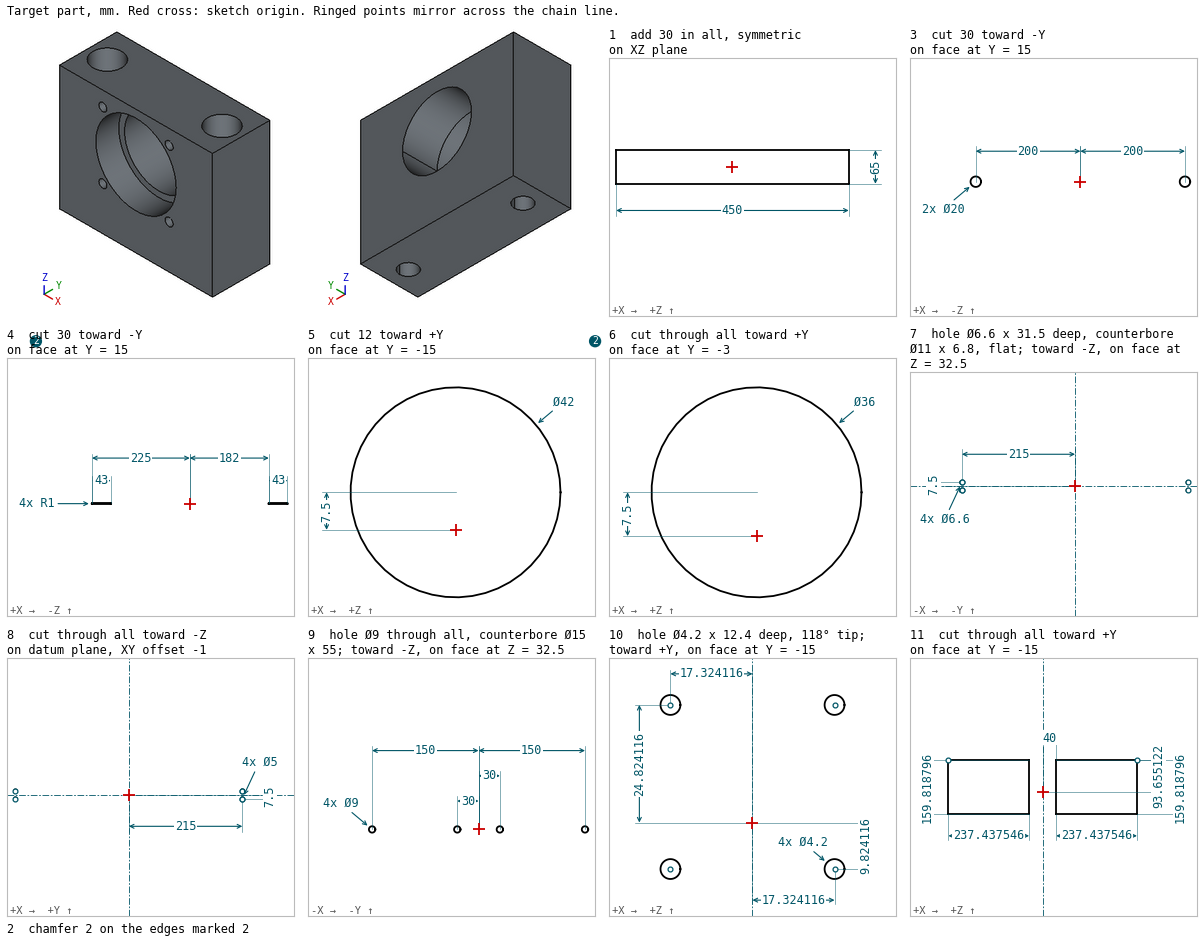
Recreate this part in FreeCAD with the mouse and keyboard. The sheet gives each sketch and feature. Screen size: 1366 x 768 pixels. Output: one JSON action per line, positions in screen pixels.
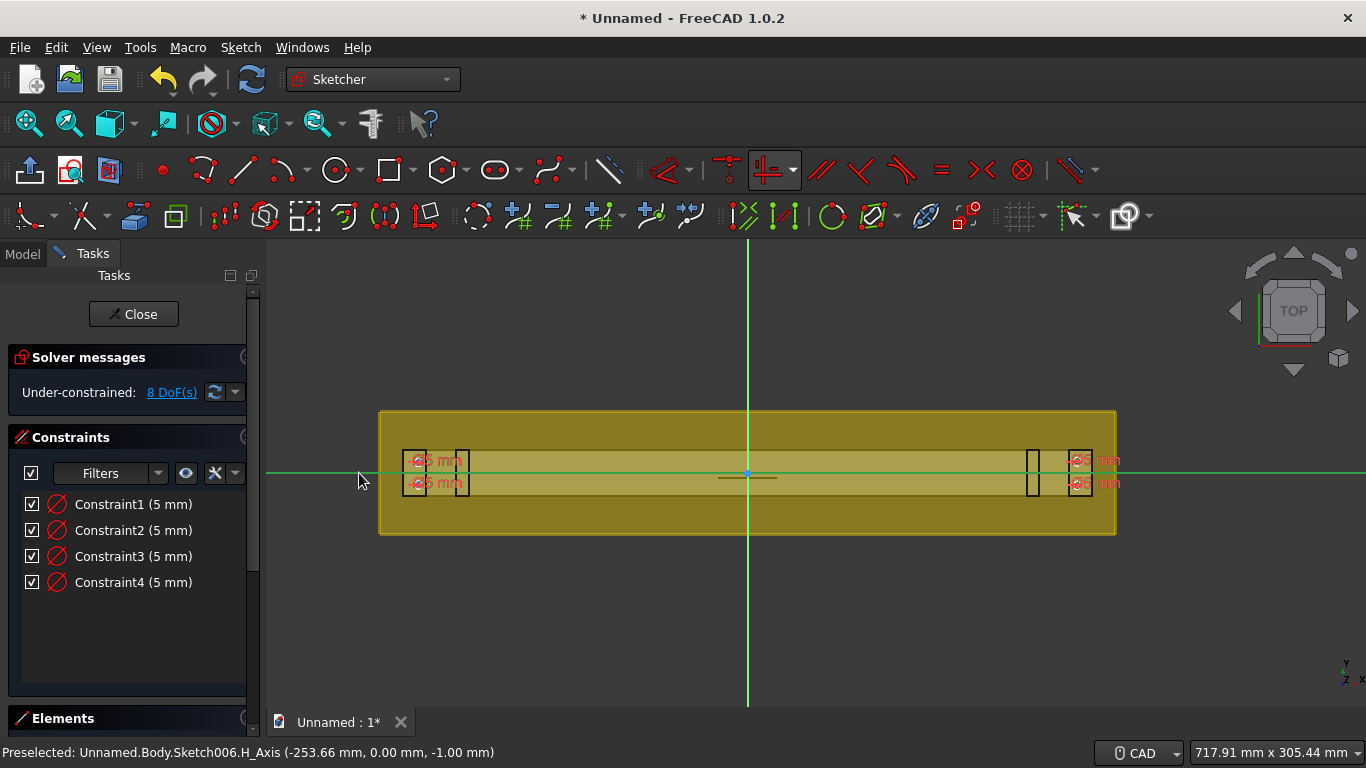
{"action": "key", "text": "s"}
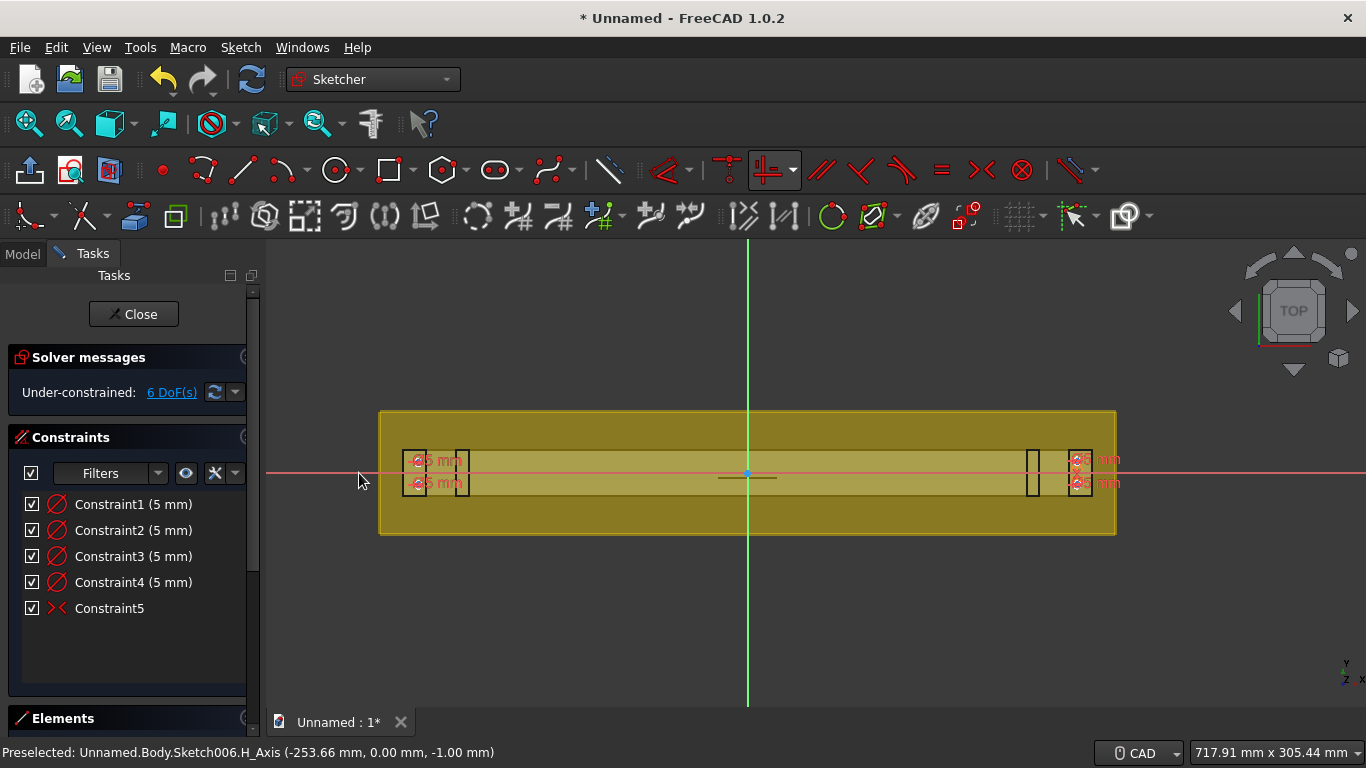
{"action": "left_click", "coordinate": [1077, 485]}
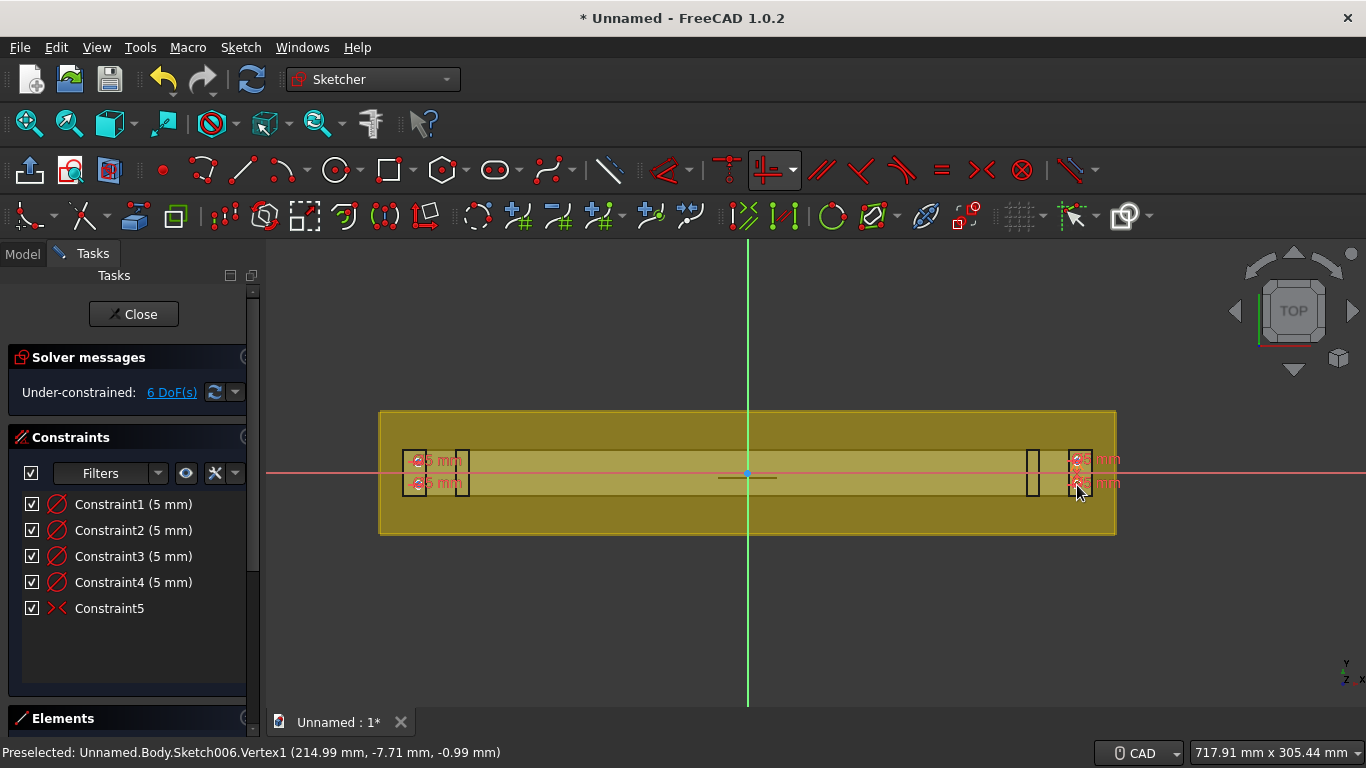
{"action": "left_click", "coordinate": [419, 485]}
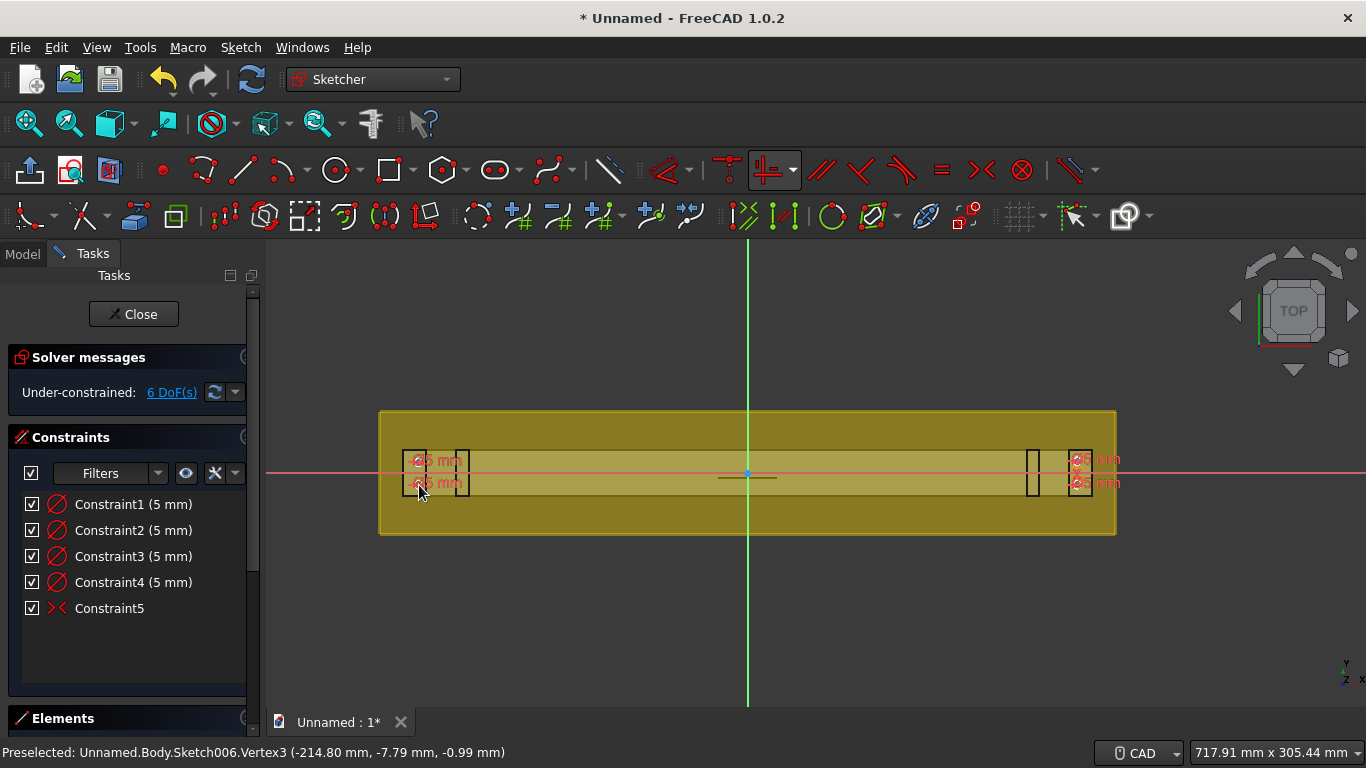
{"action": "left_click", "coordinate": [748, 650]}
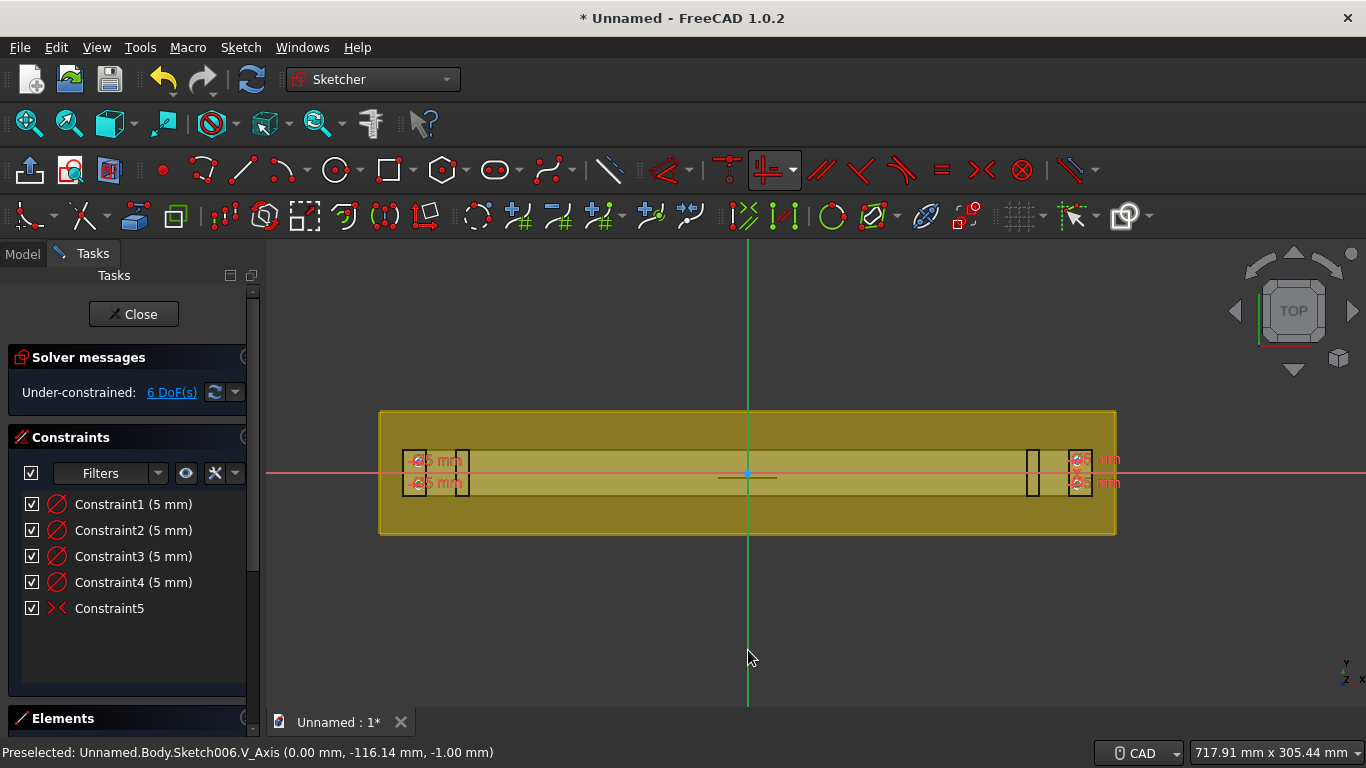
{"action": "left_click", "coordinate": [982, 170]}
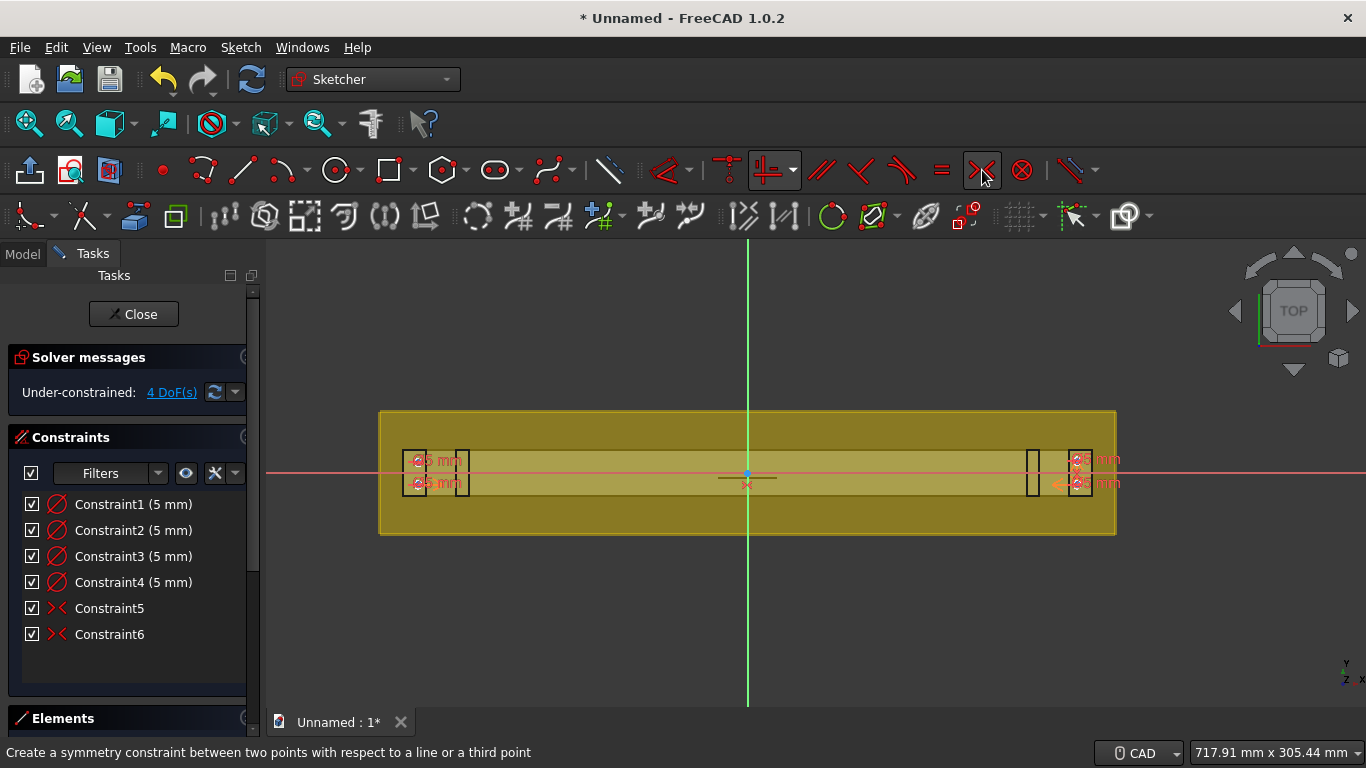
{"action": "left_click", "coordinate": [1077, 461]}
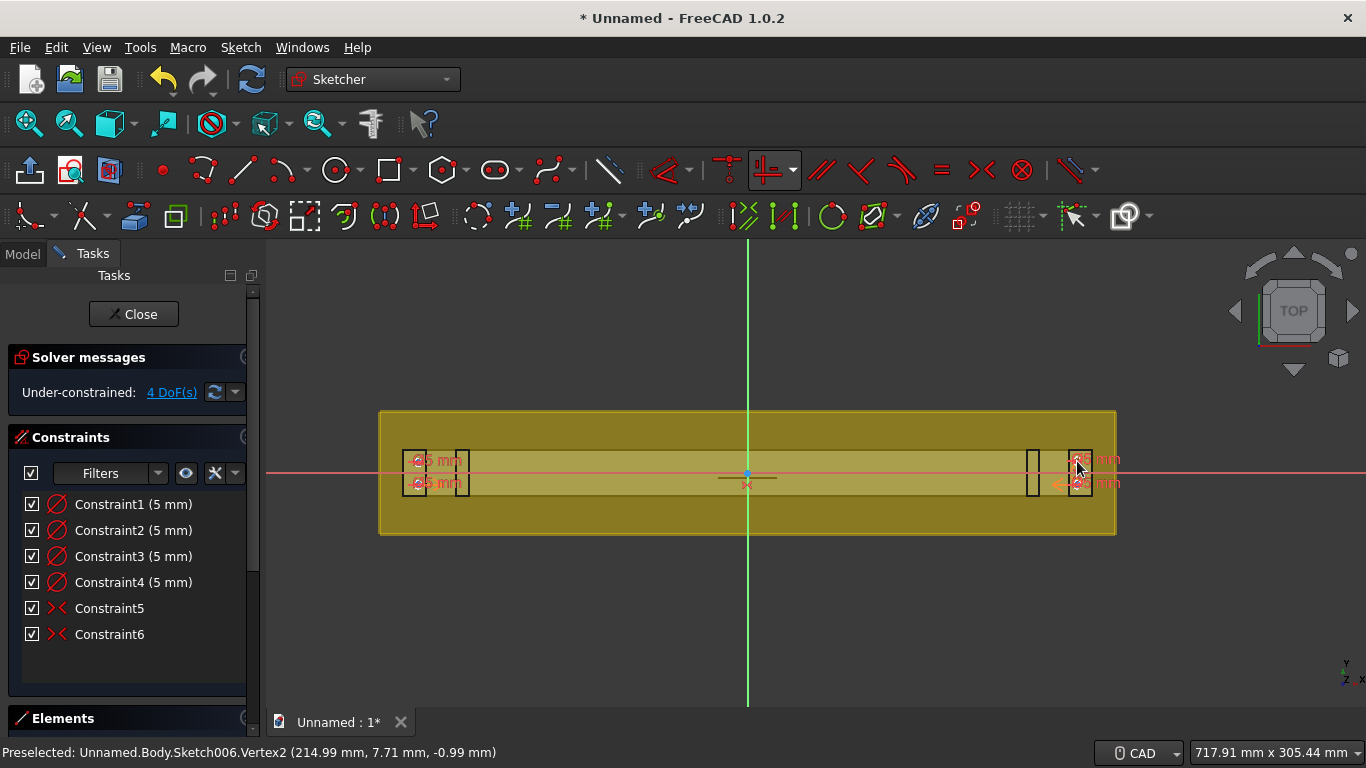
{"action": "left_click", "coordinate": [418, 462]}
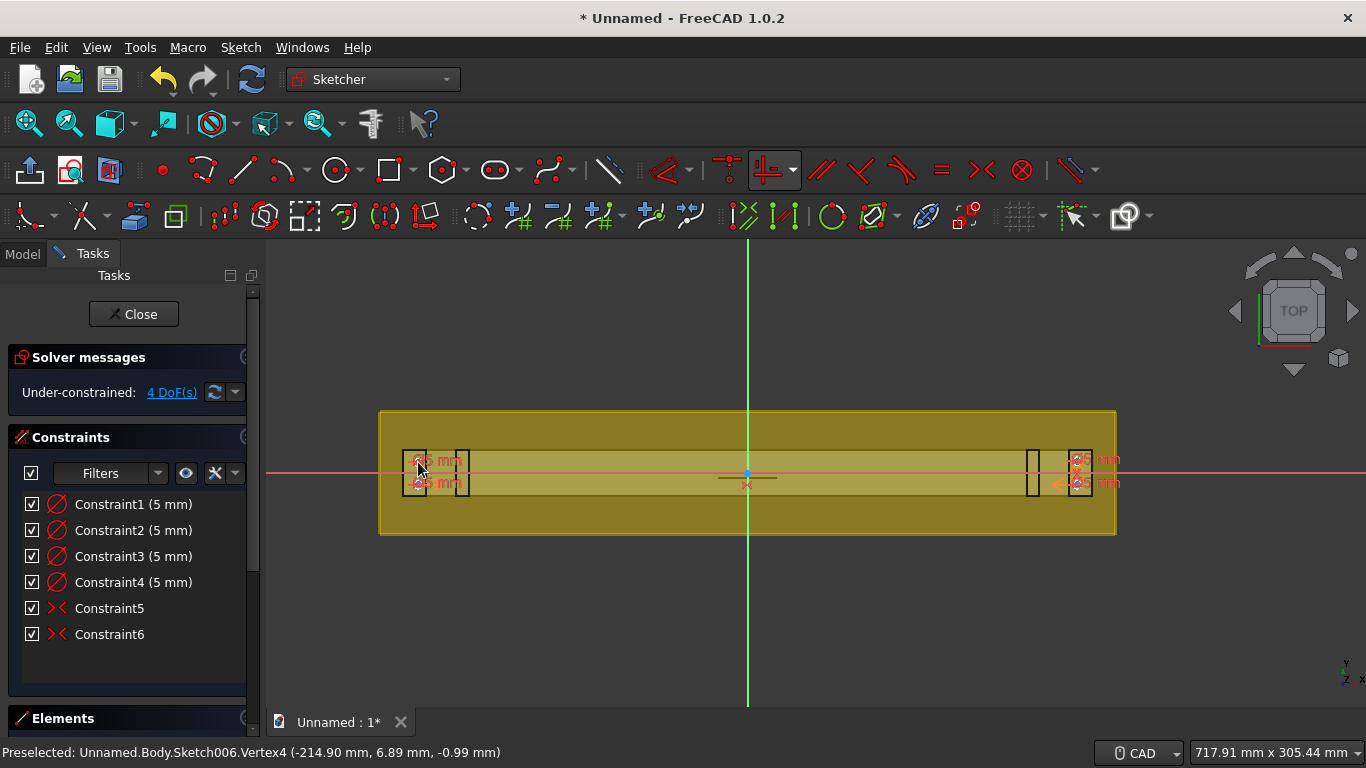
{"action": "left_click", "coordinate": [748, 650]}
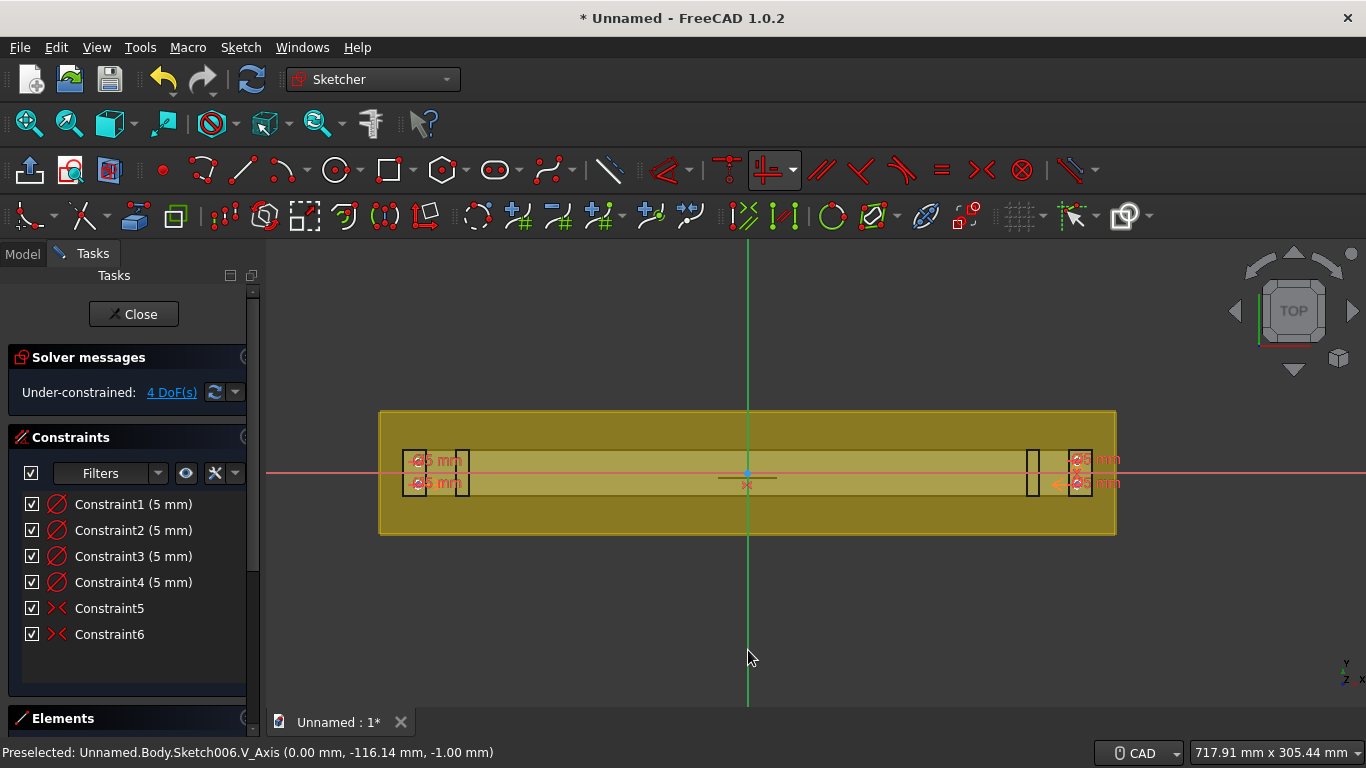
{"action": "key", "text": "s"}